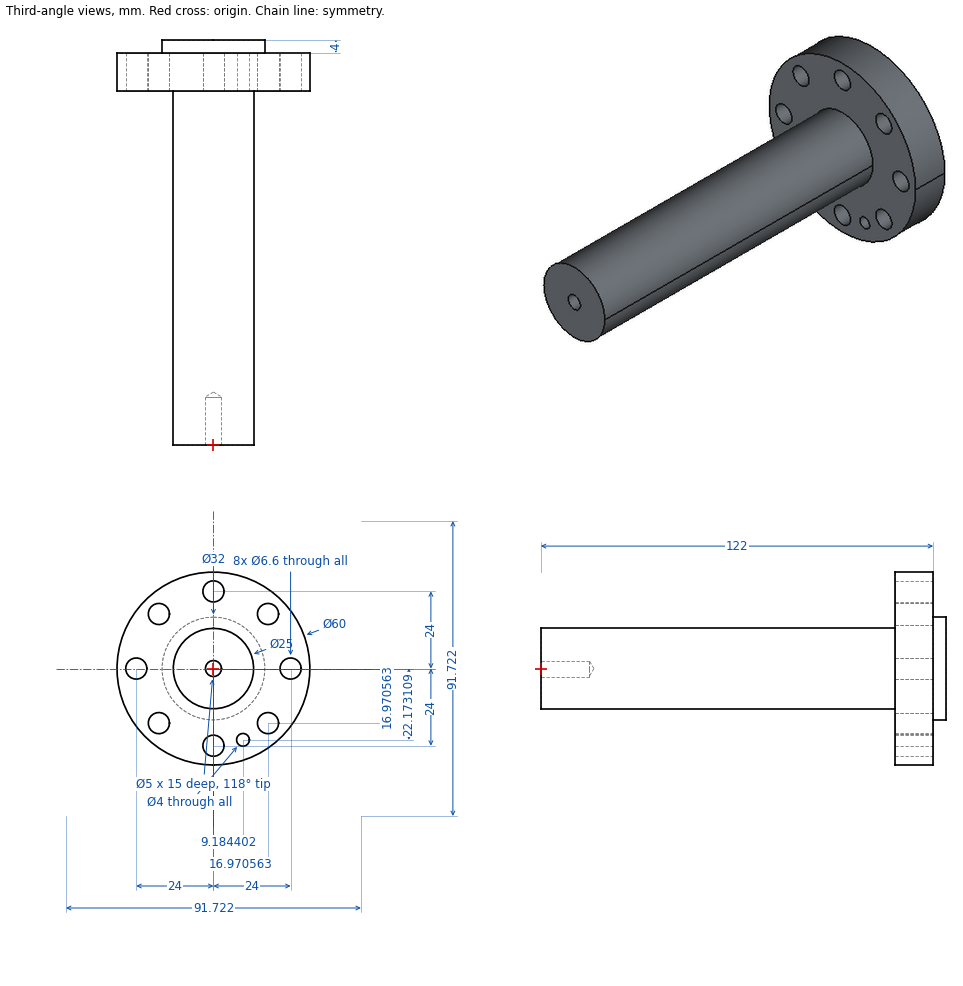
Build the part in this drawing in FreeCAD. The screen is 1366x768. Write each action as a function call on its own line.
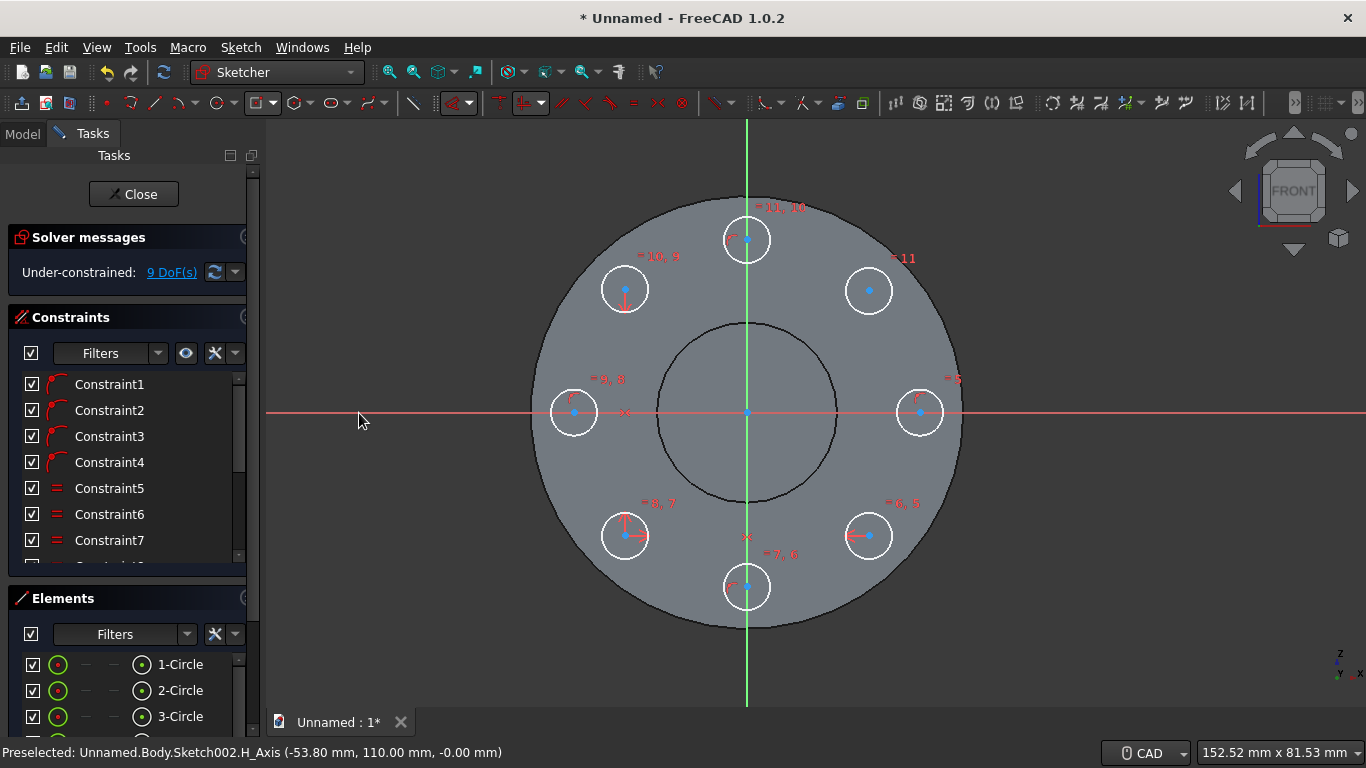
click(869, 536)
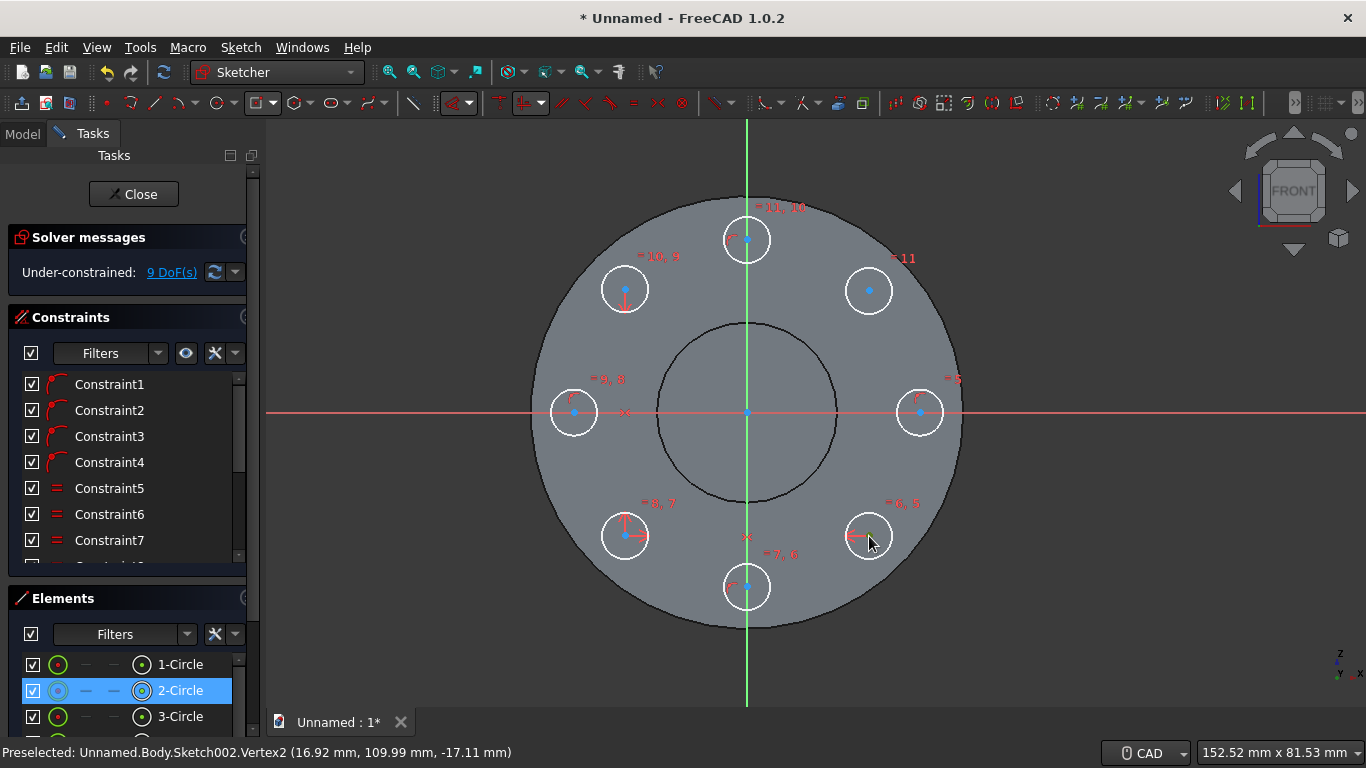
click(869, 291)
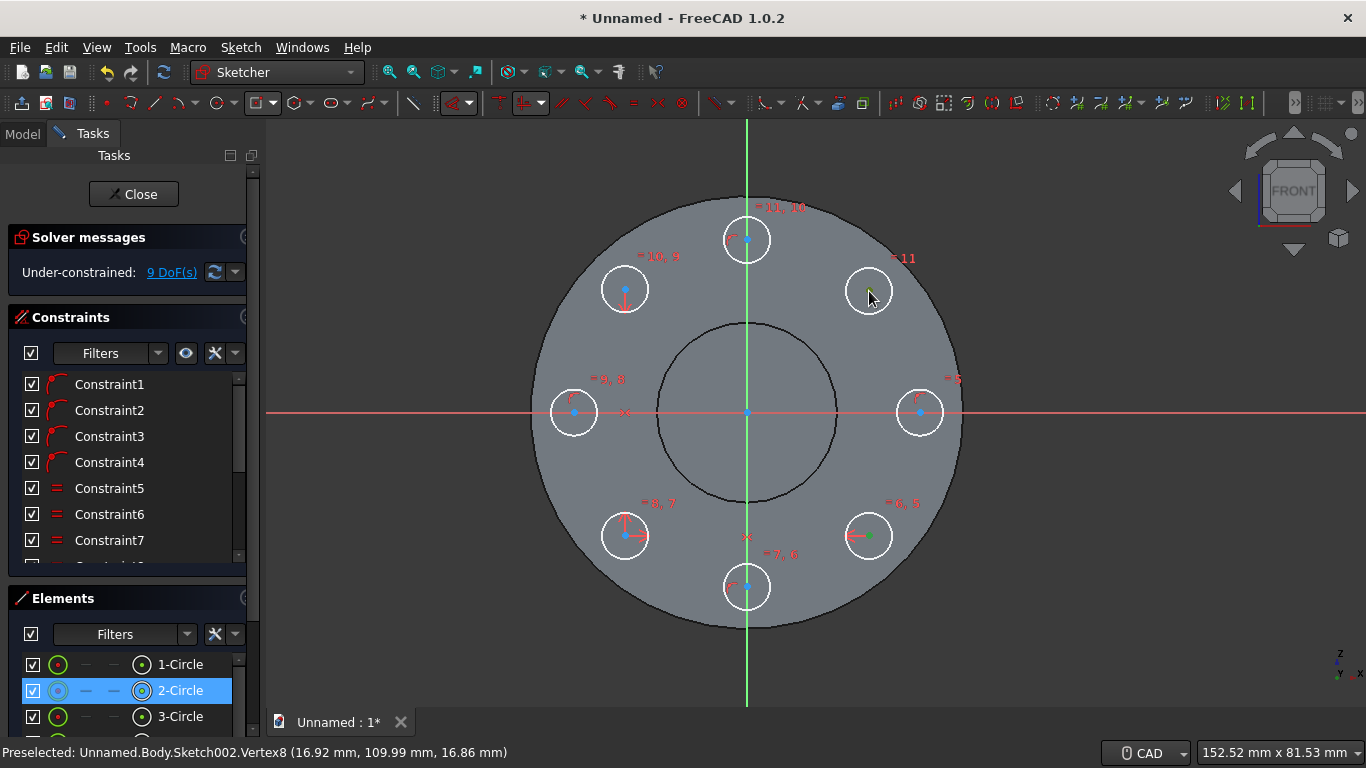
click(359, 413)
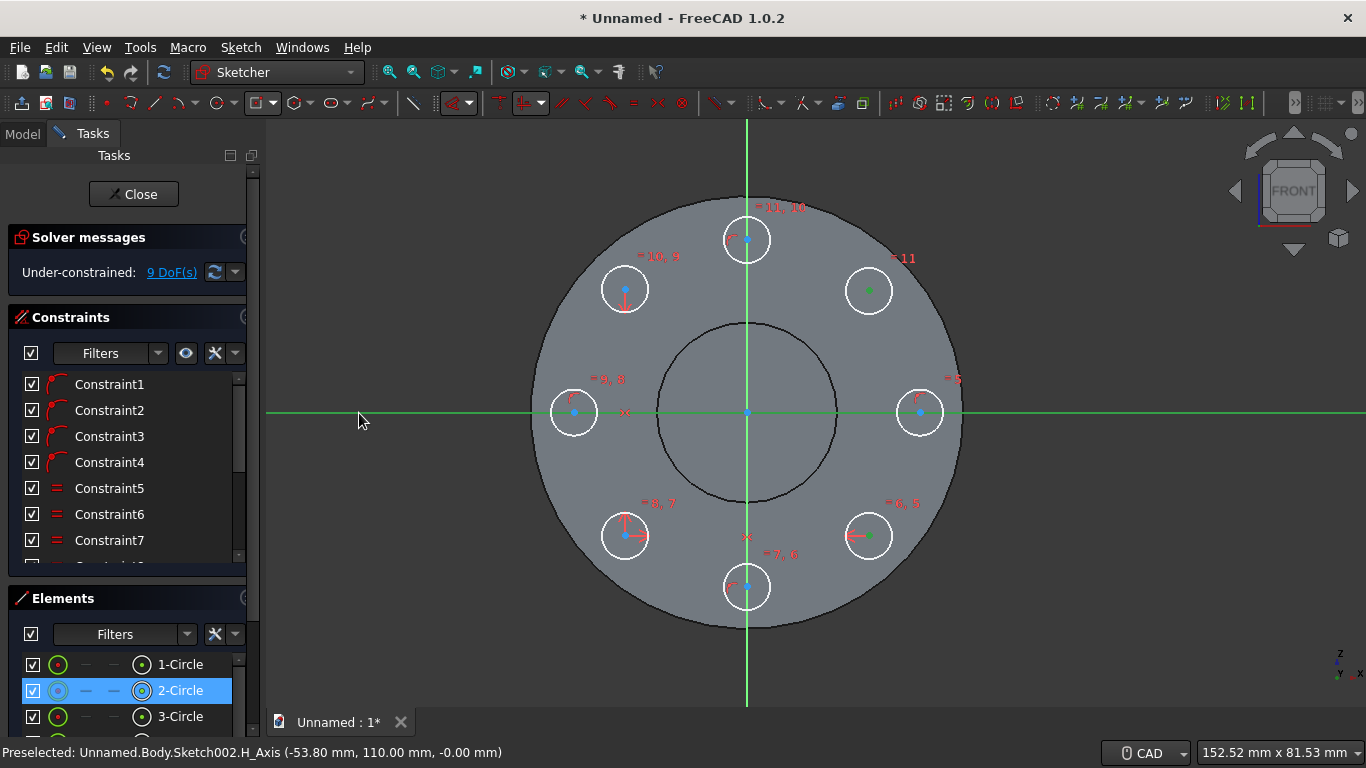
click(658, 104)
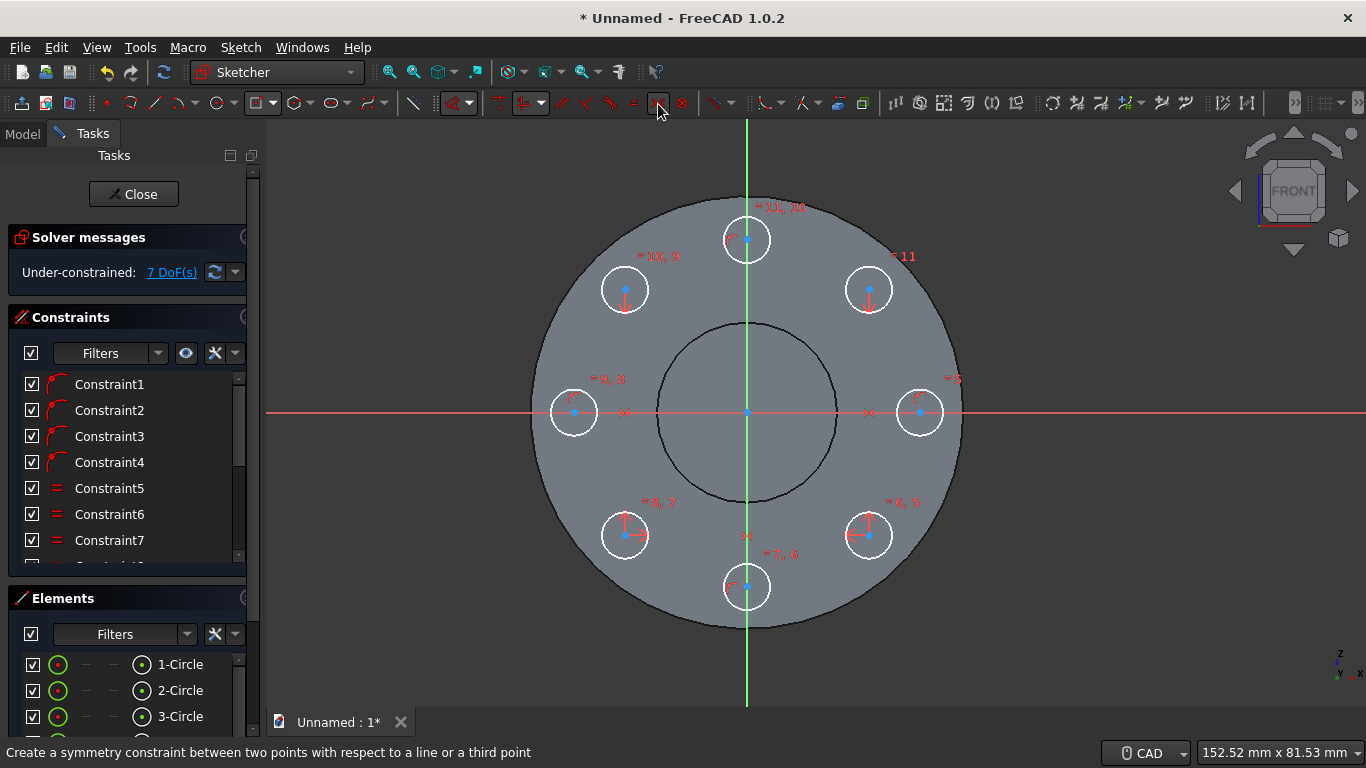
click(936, 396)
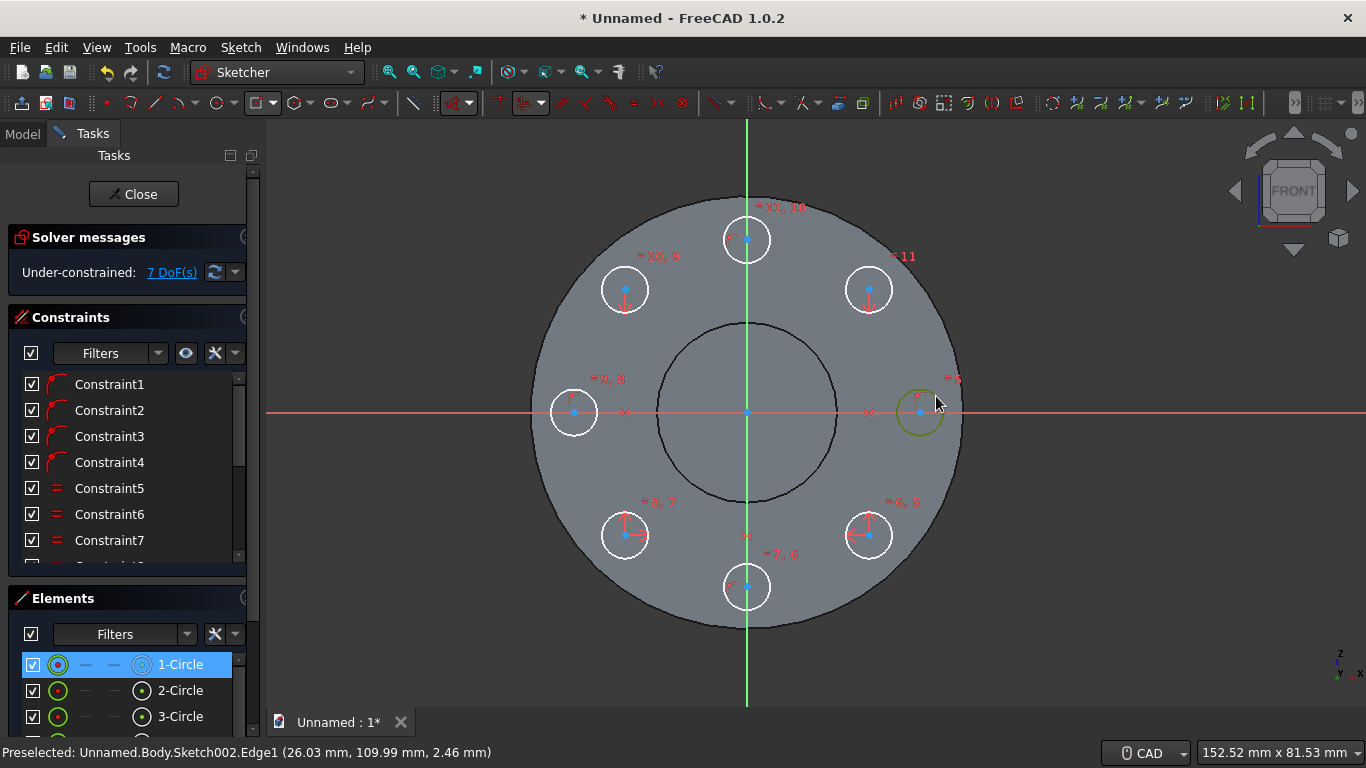
click(472, 104)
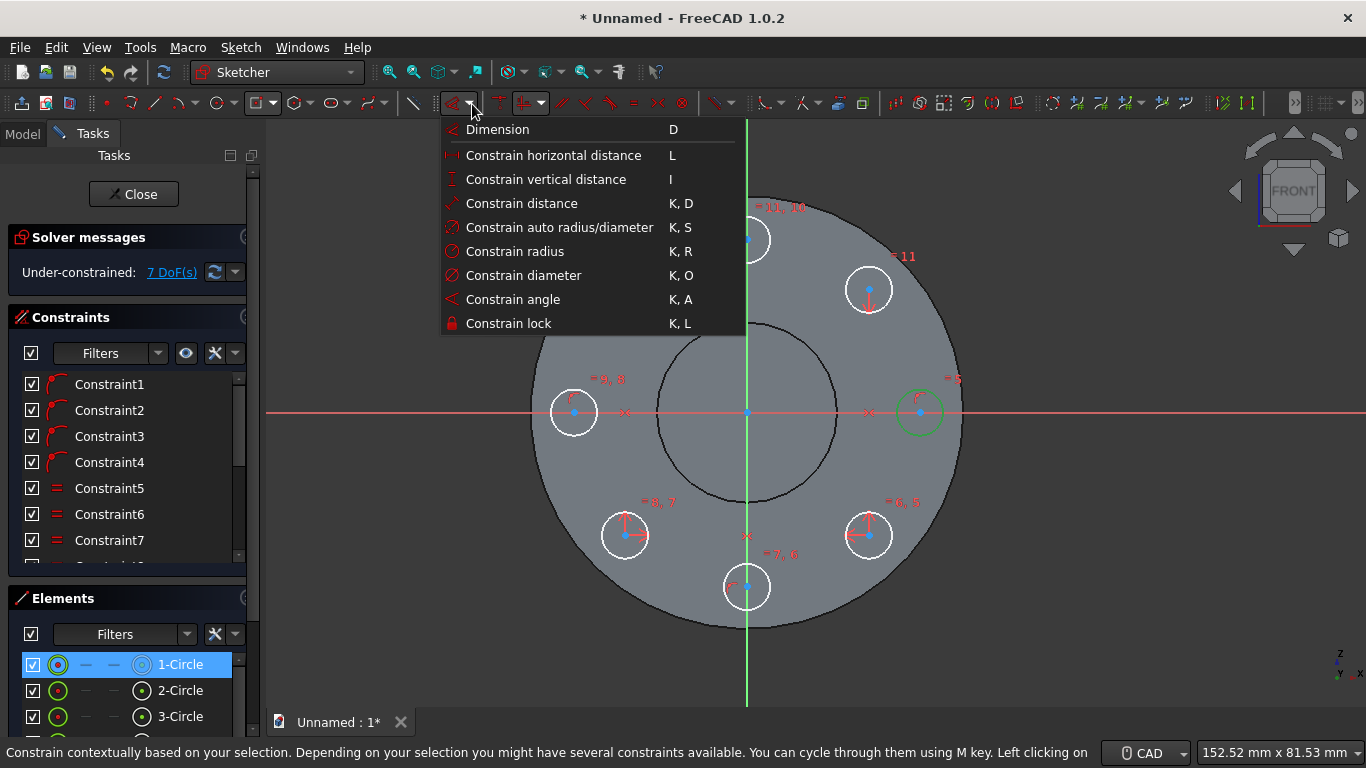
click(593, 275)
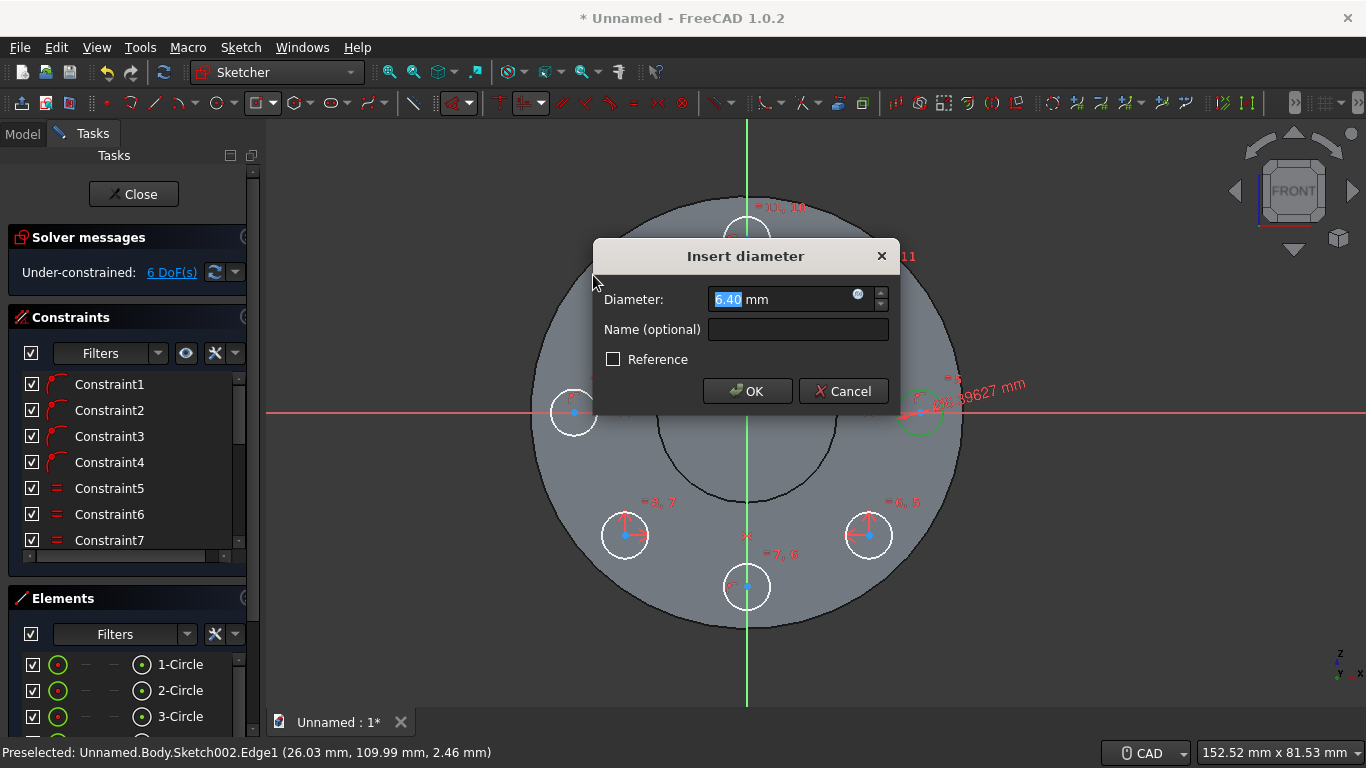
text(6.6)
key(Return)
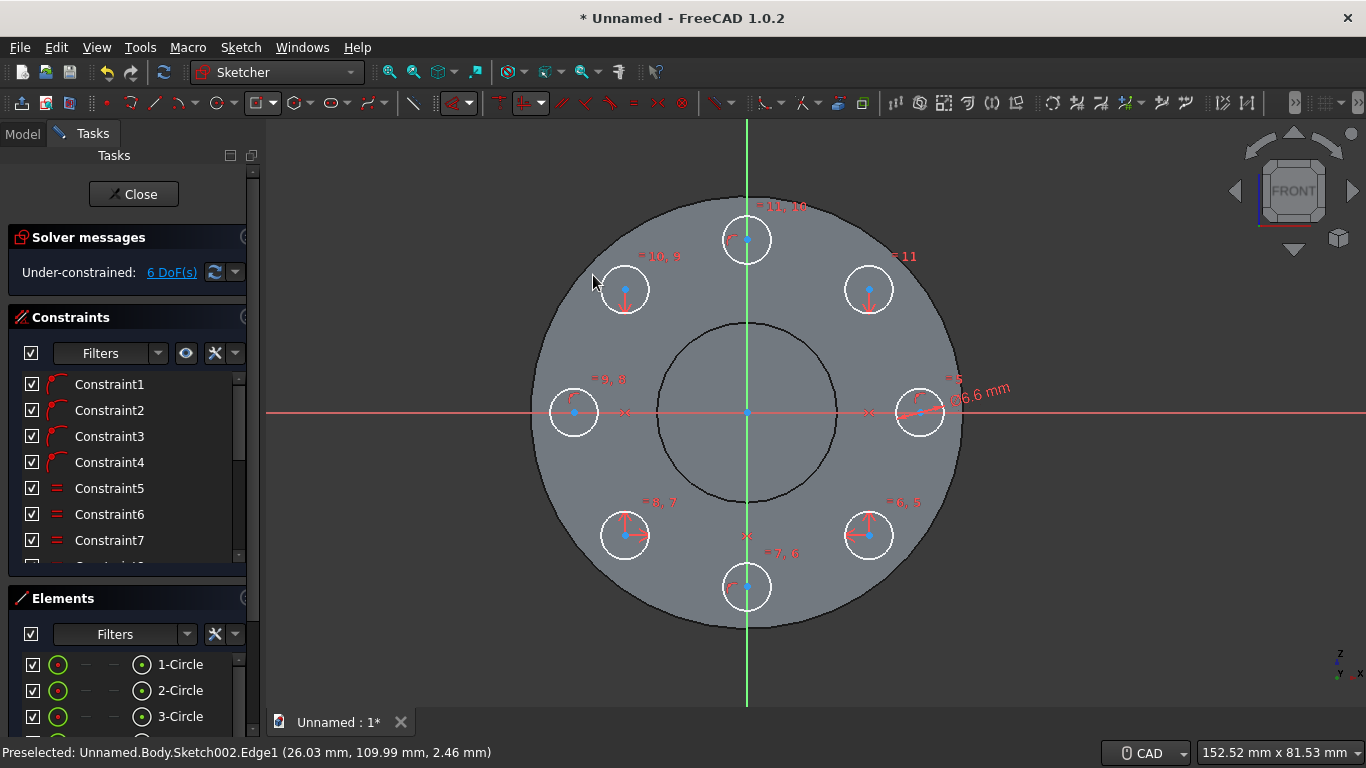
click(920, 413)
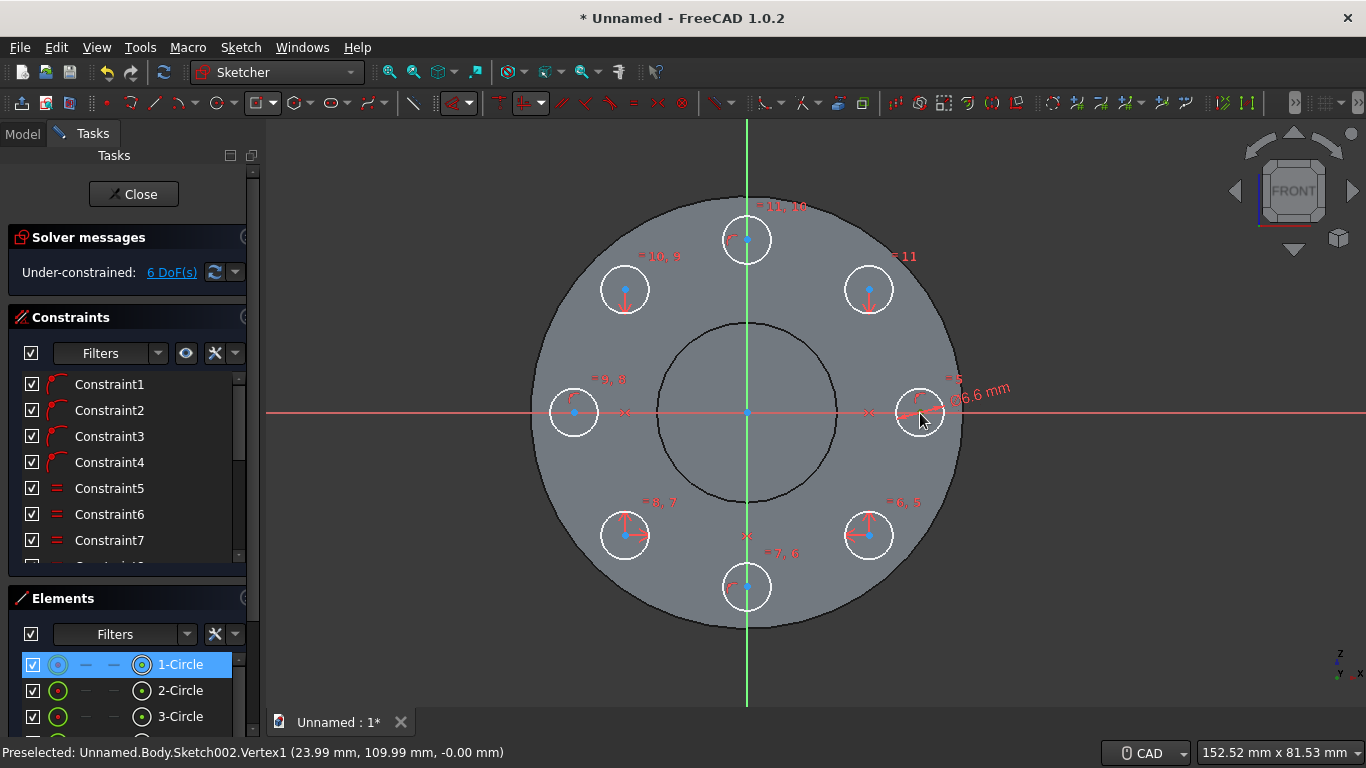
key(l)